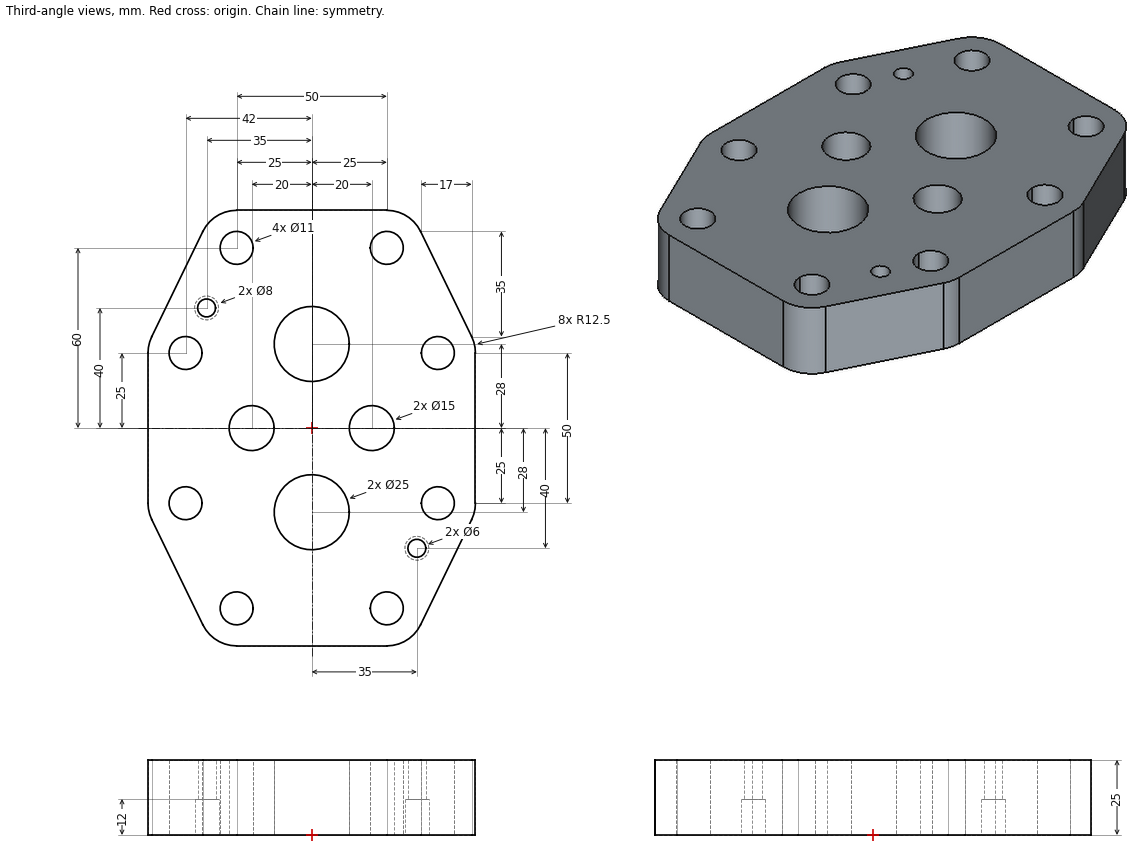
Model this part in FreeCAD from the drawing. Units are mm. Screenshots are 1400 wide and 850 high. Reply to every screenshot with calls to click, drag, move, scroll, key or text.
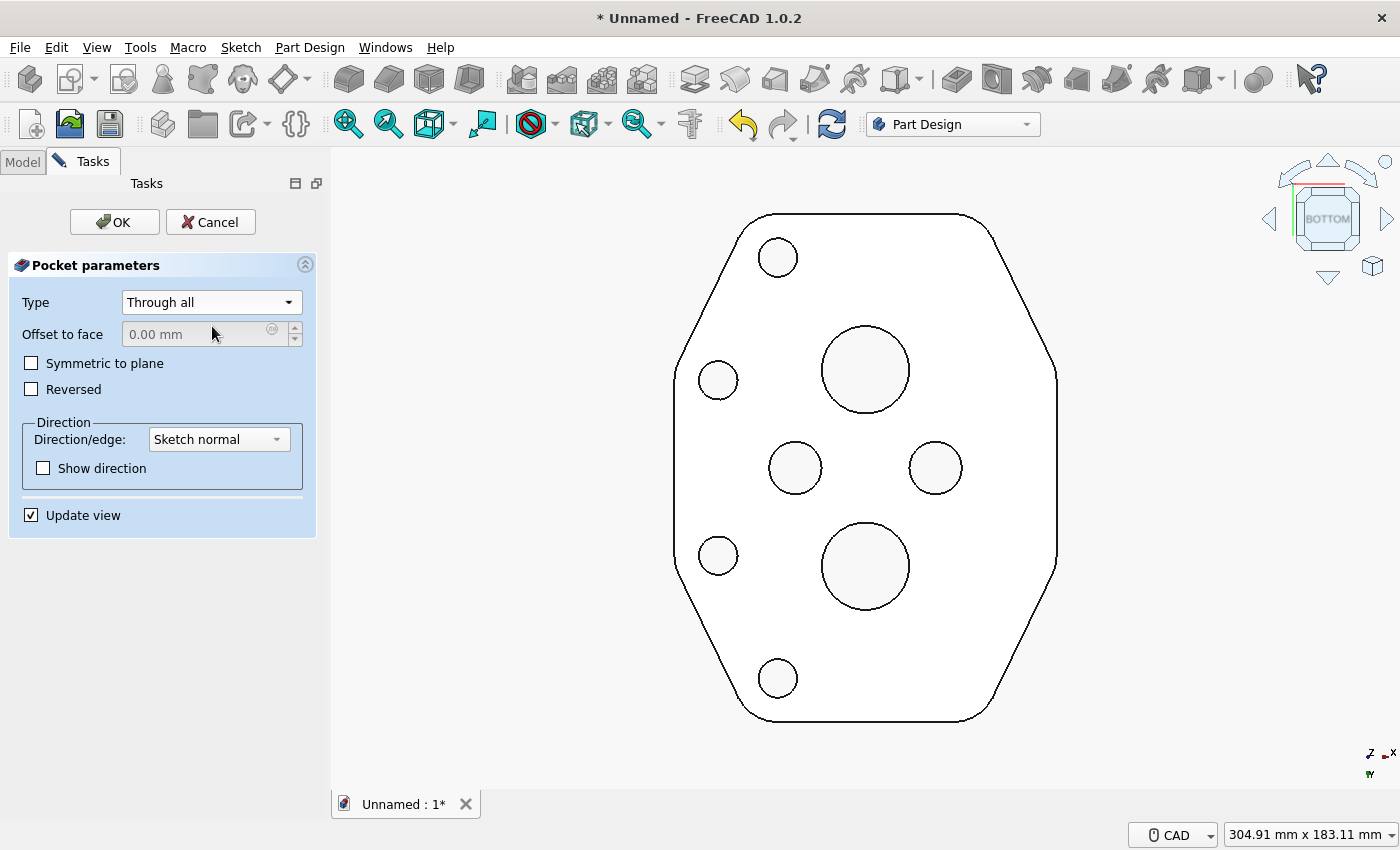
click(115, 222)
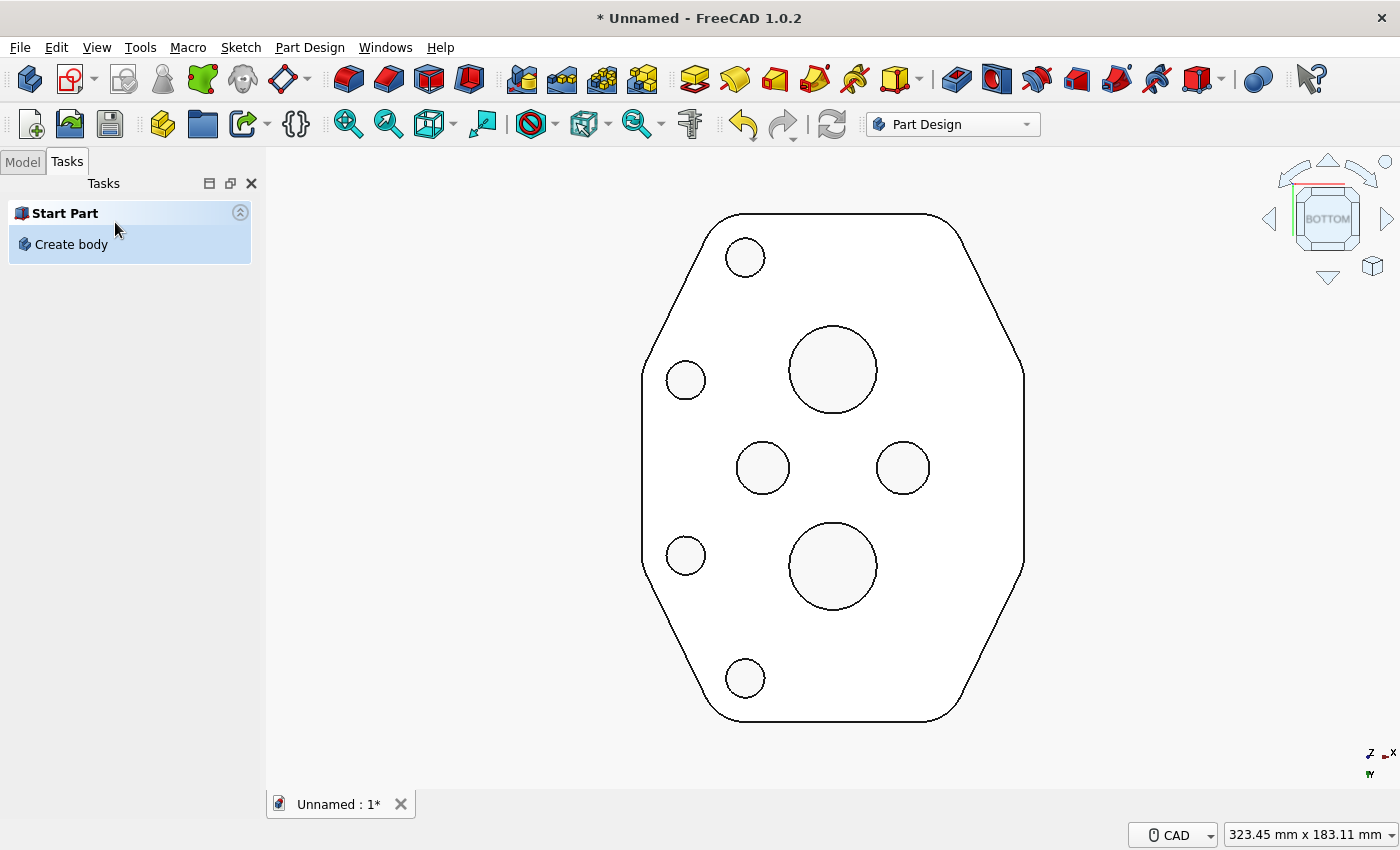
click(23, 161)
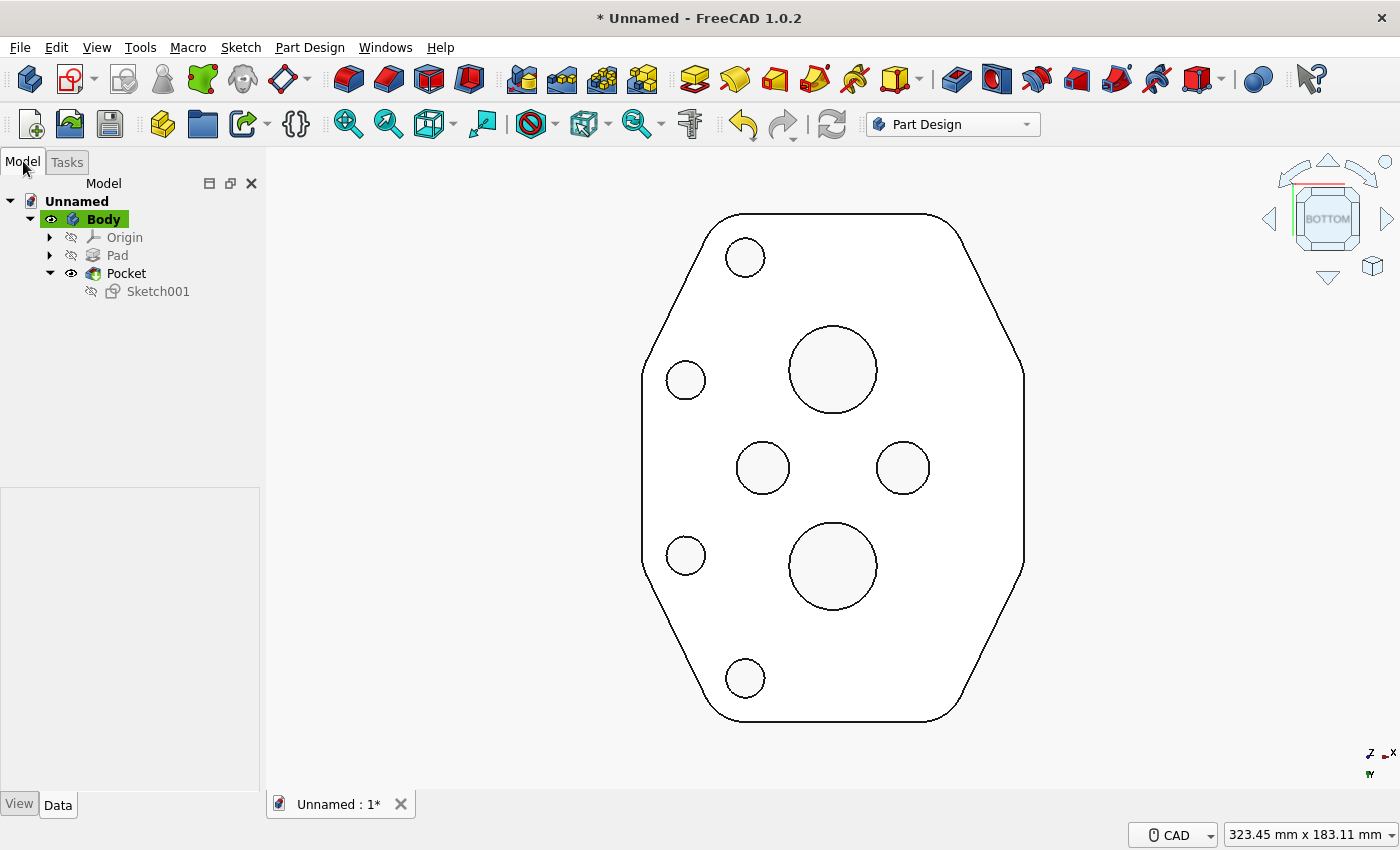
click(116, 273)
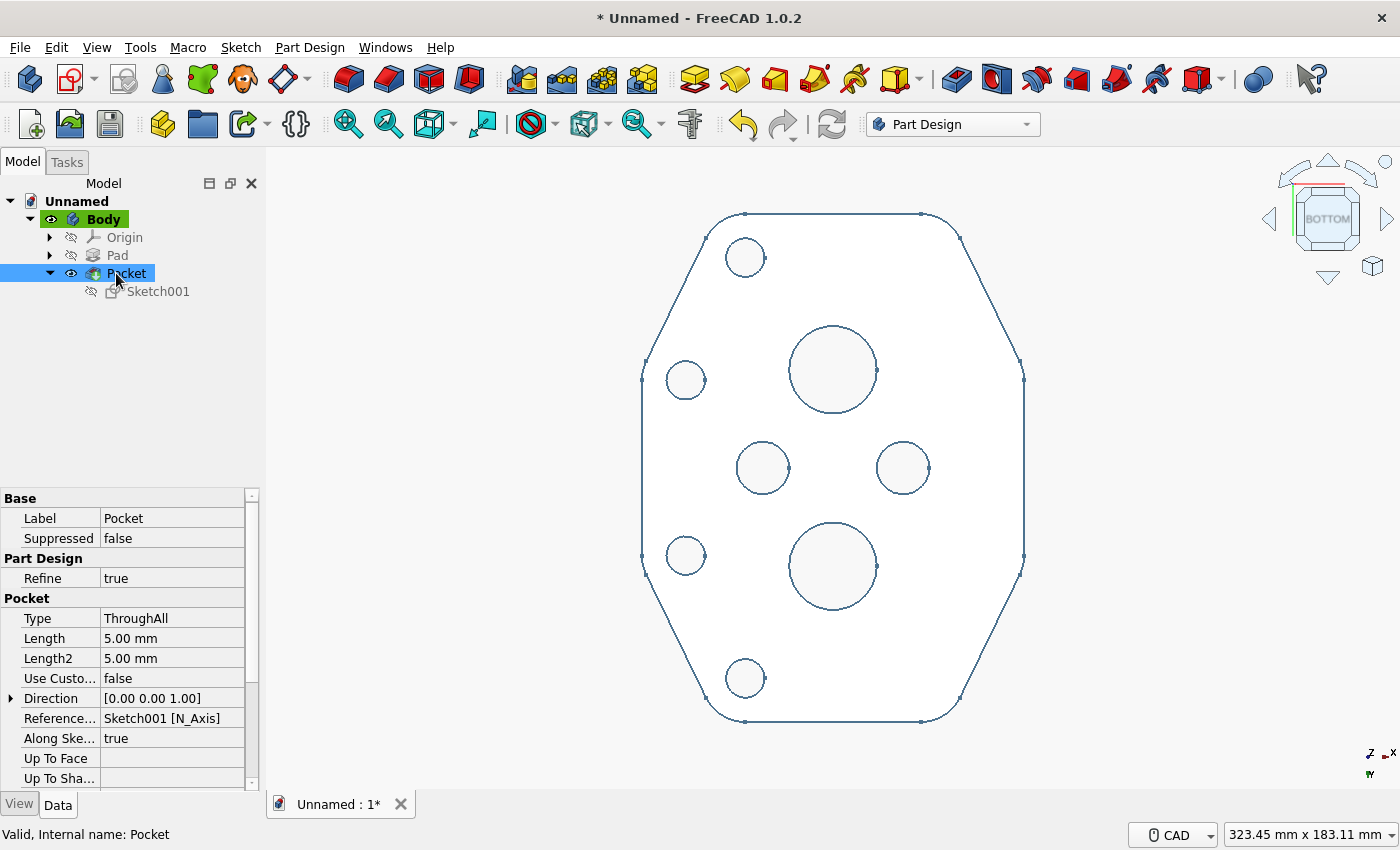
click(522, 80)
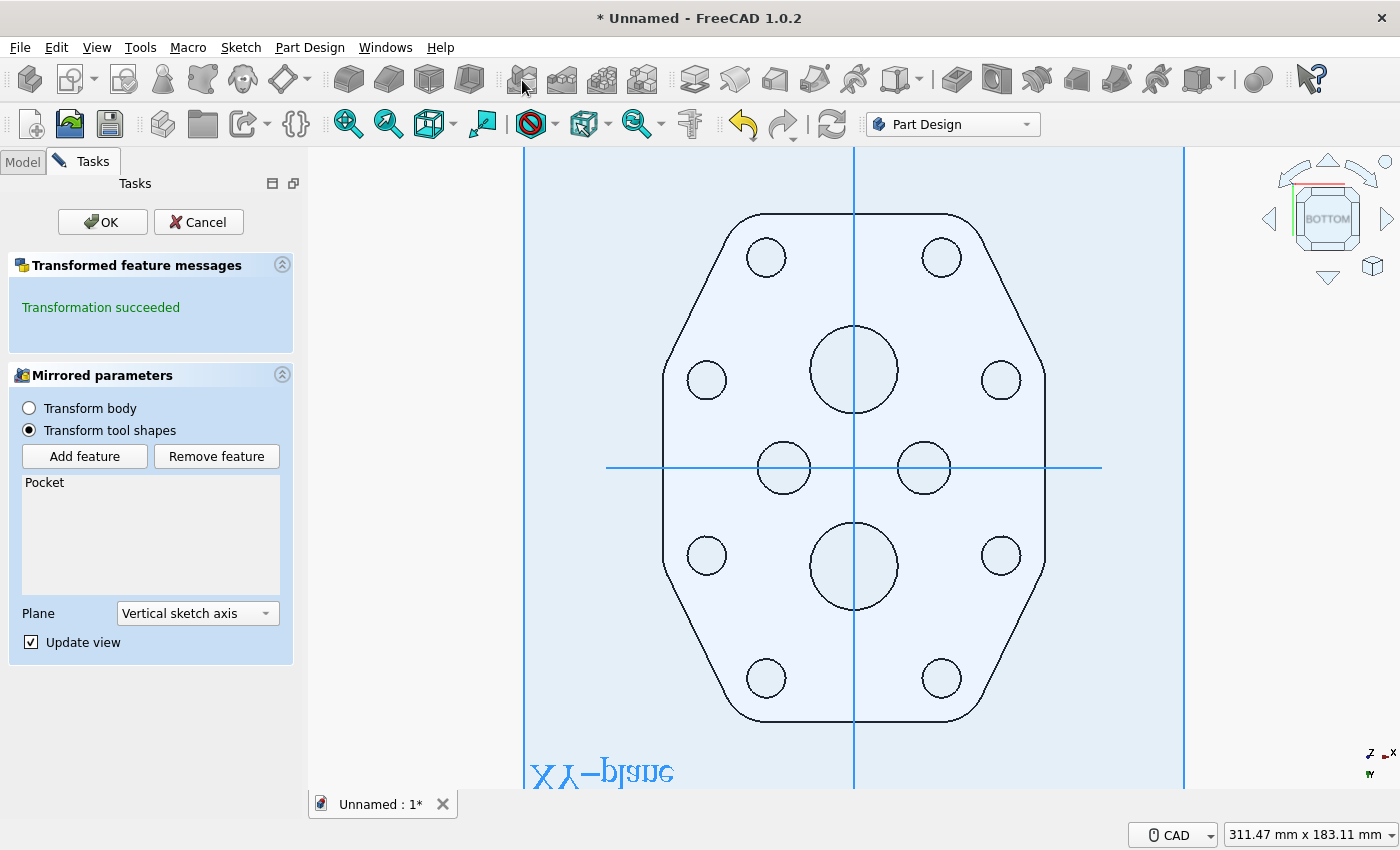
click(198, 614)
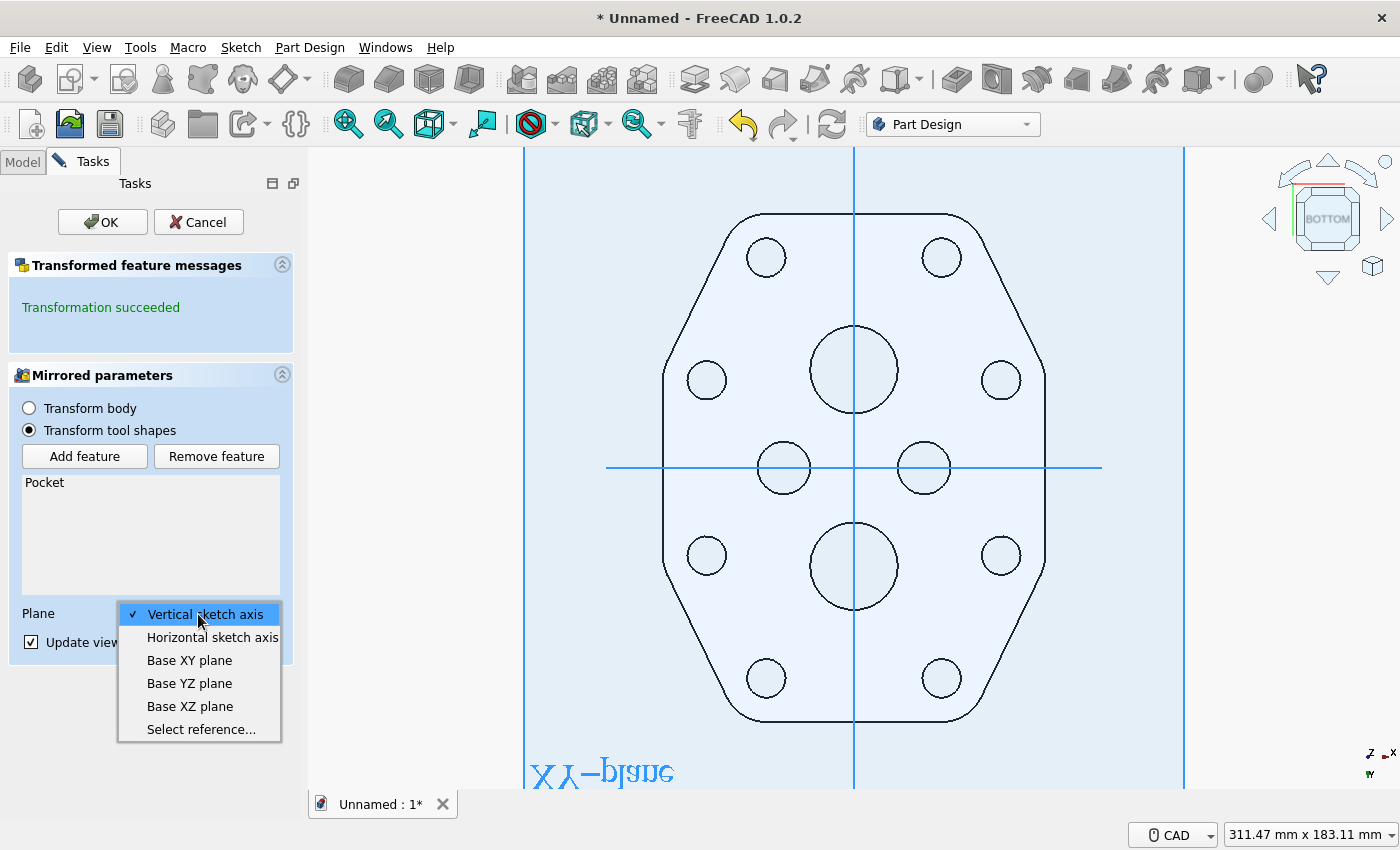
click(198, 684)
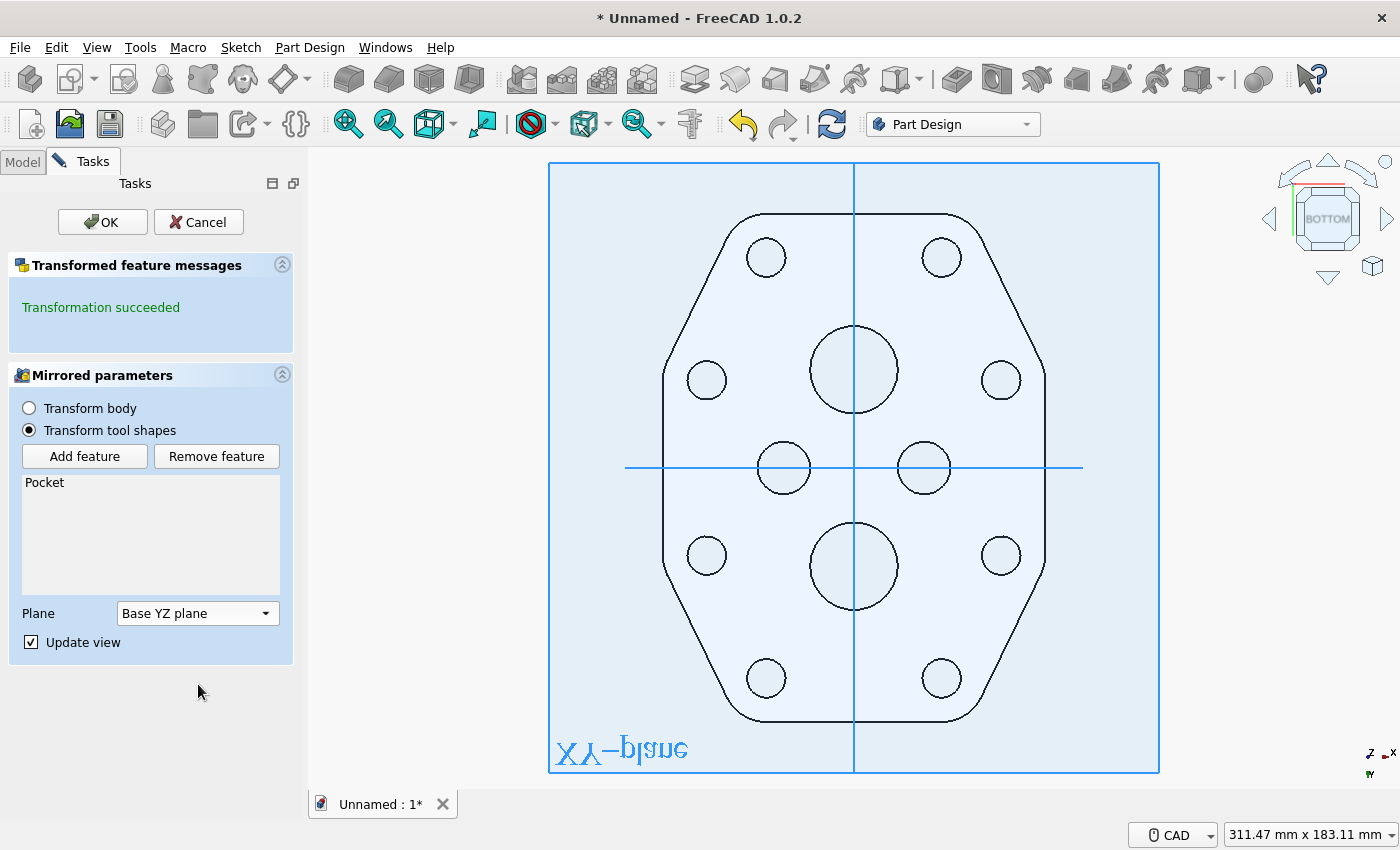
click(103, 222)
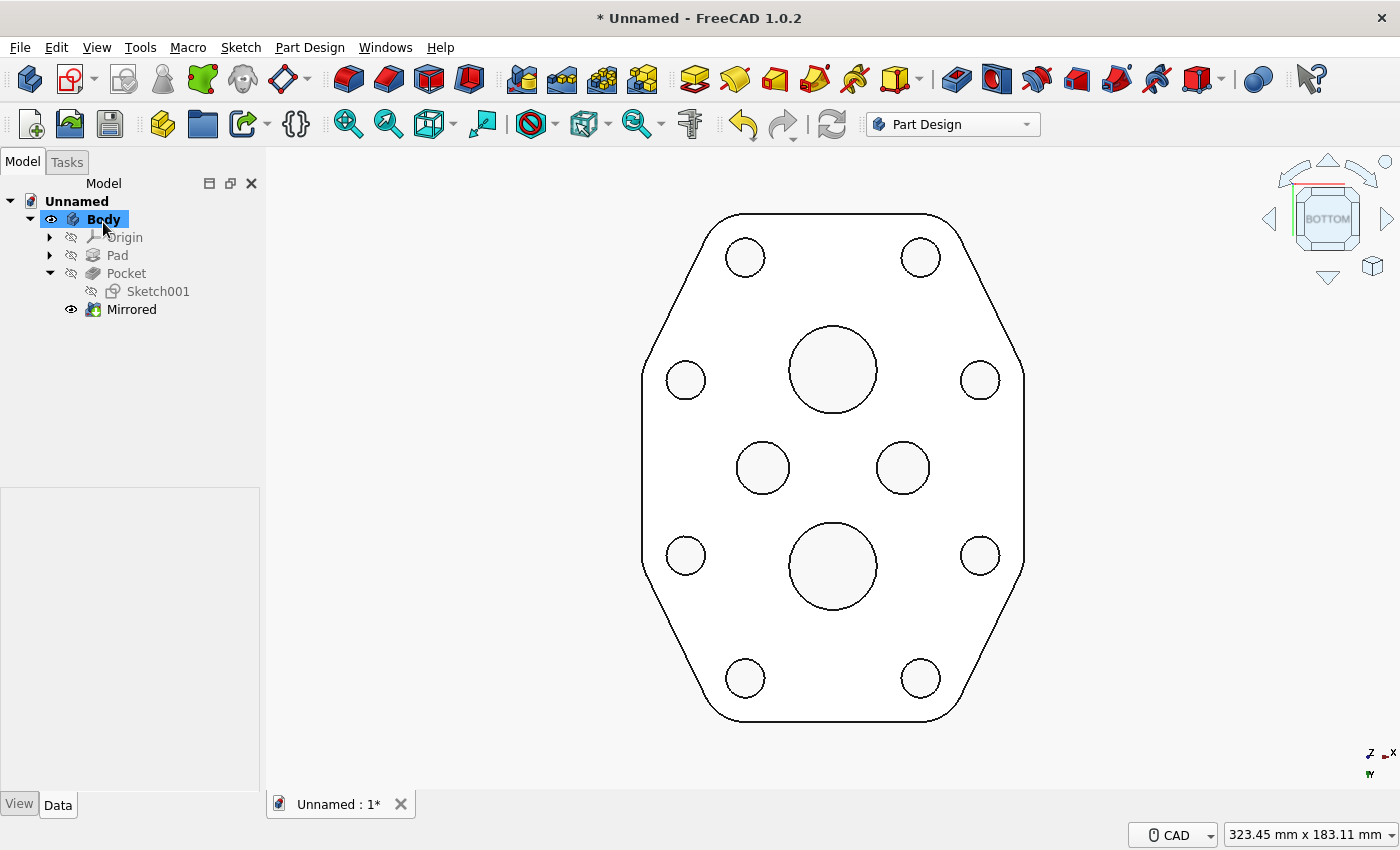
click(70, 80)